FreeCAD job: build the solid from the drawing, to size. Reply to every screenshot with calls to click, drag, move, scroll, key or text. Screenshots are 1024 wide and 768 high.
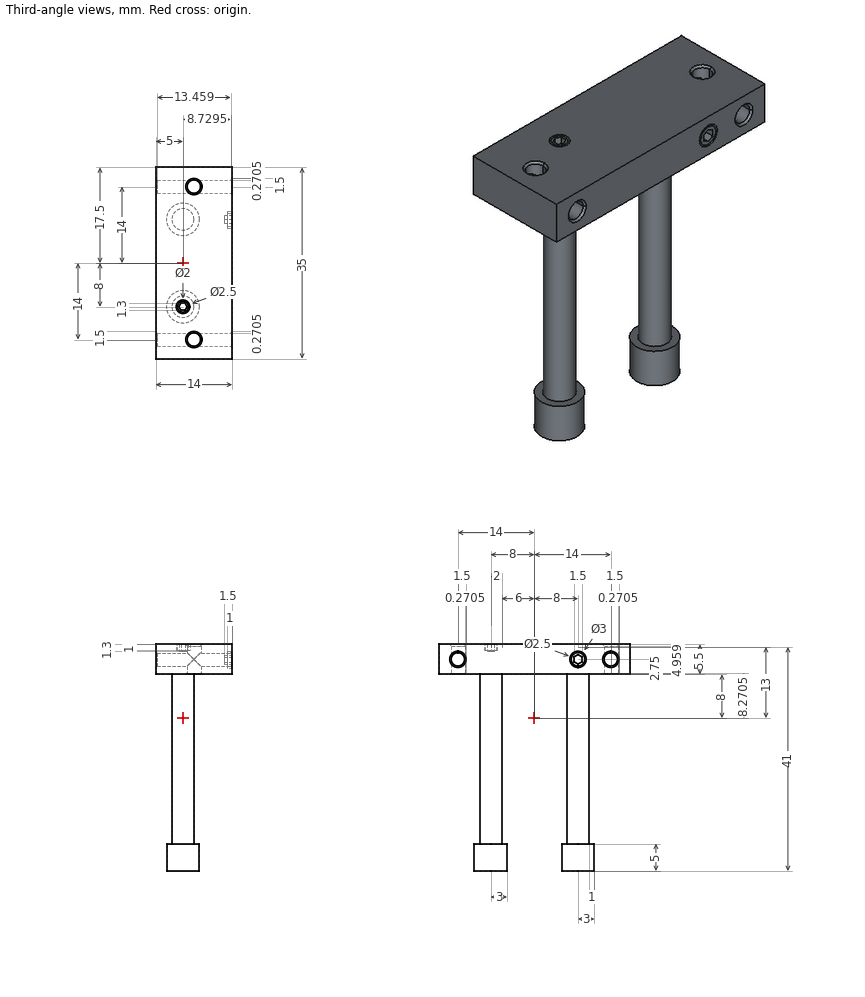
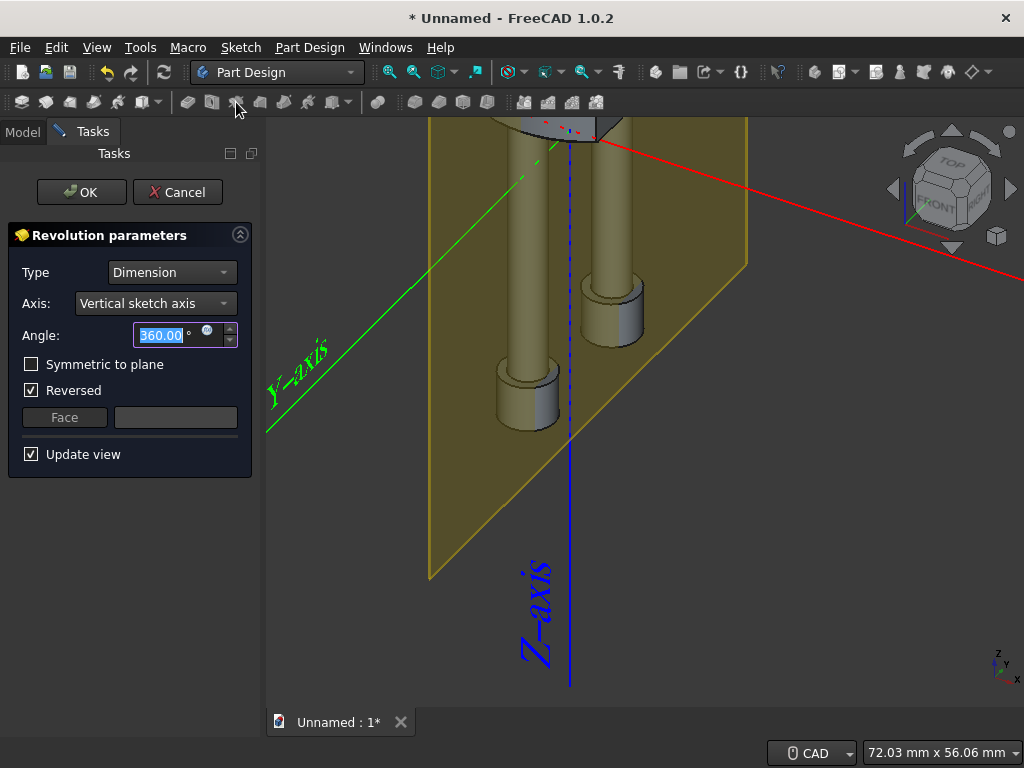
click(156, 304)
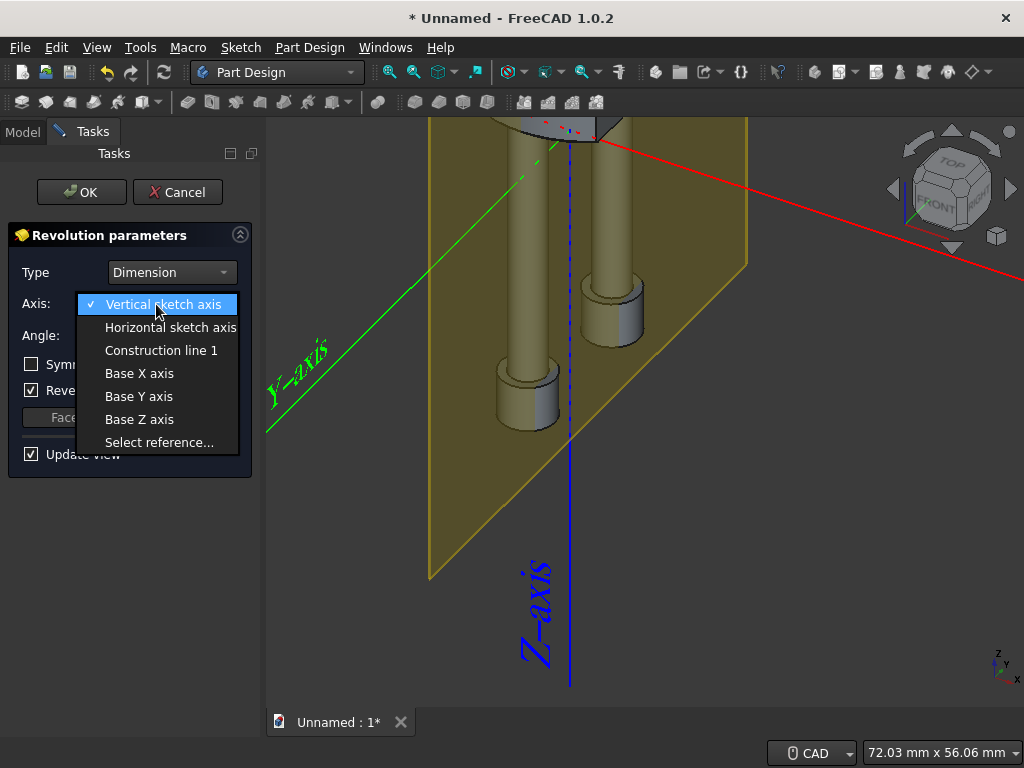
click(156, 350)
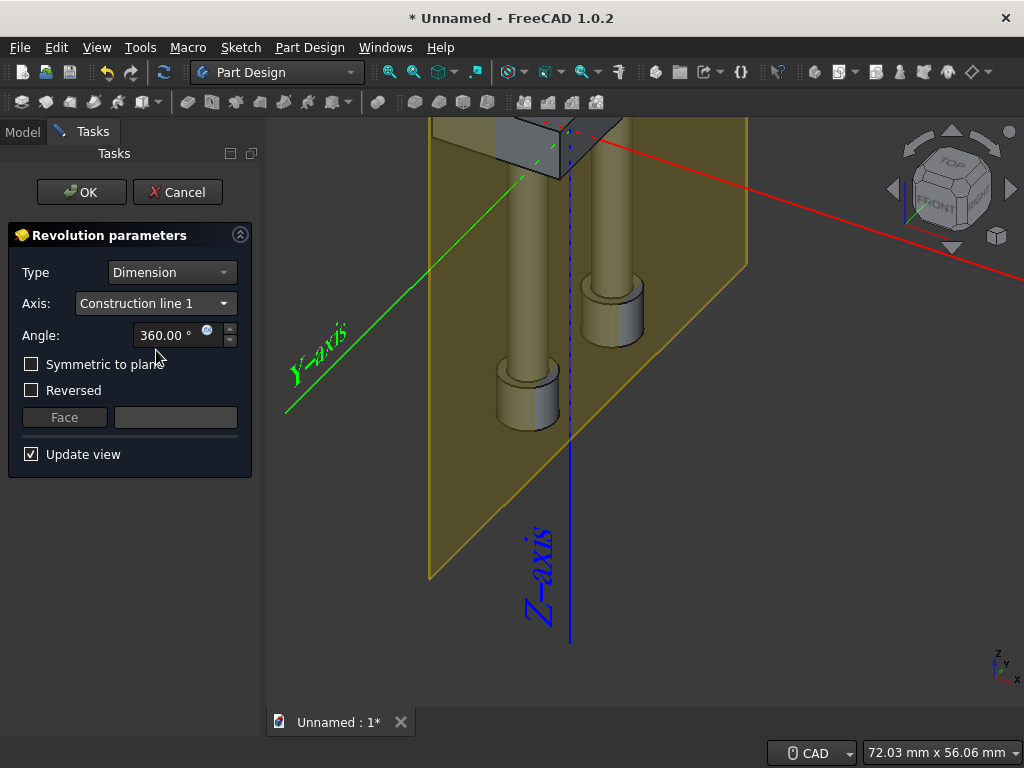
click(82, 192)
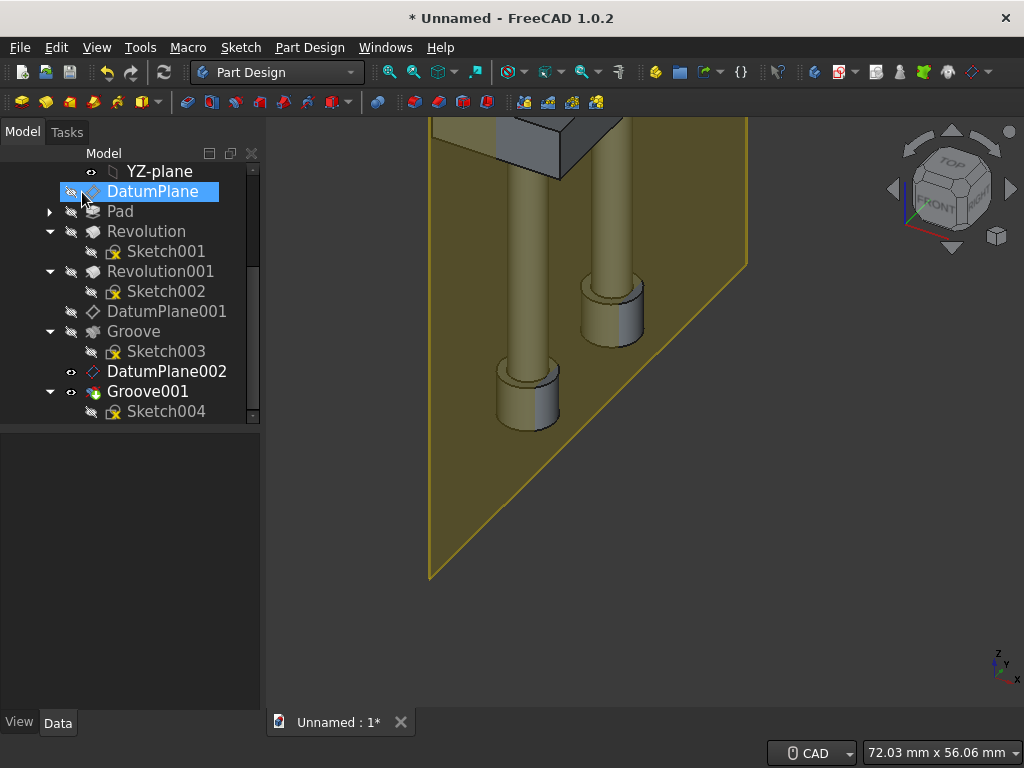
click(116, 372)
key(space)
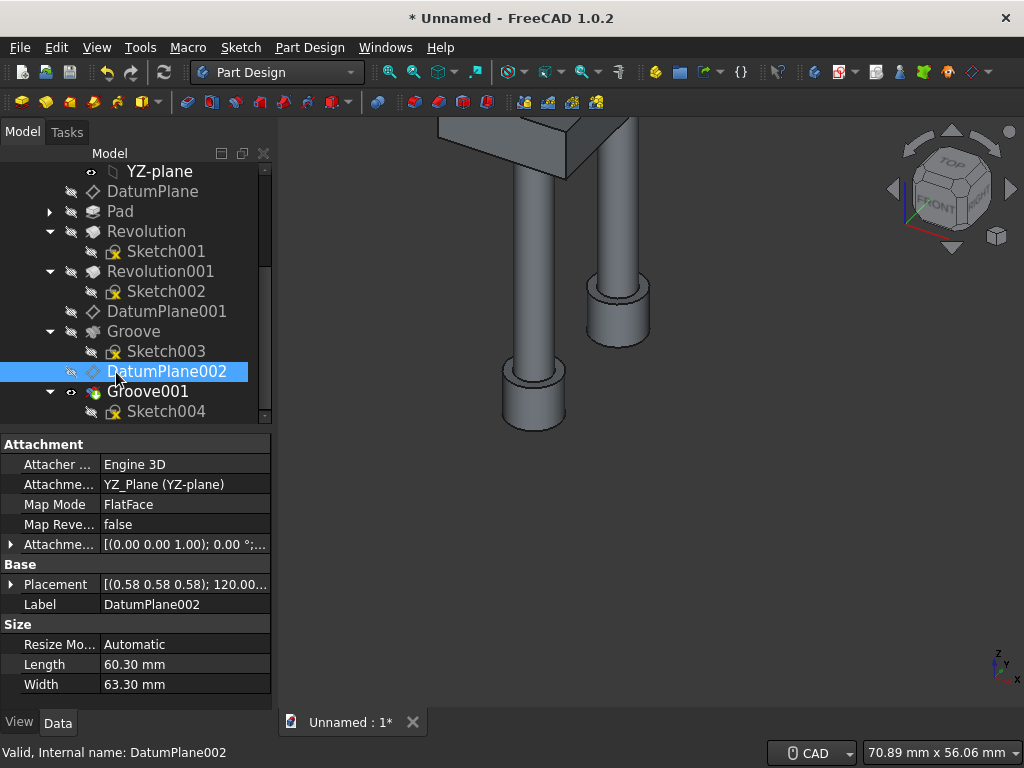
click(390, 72)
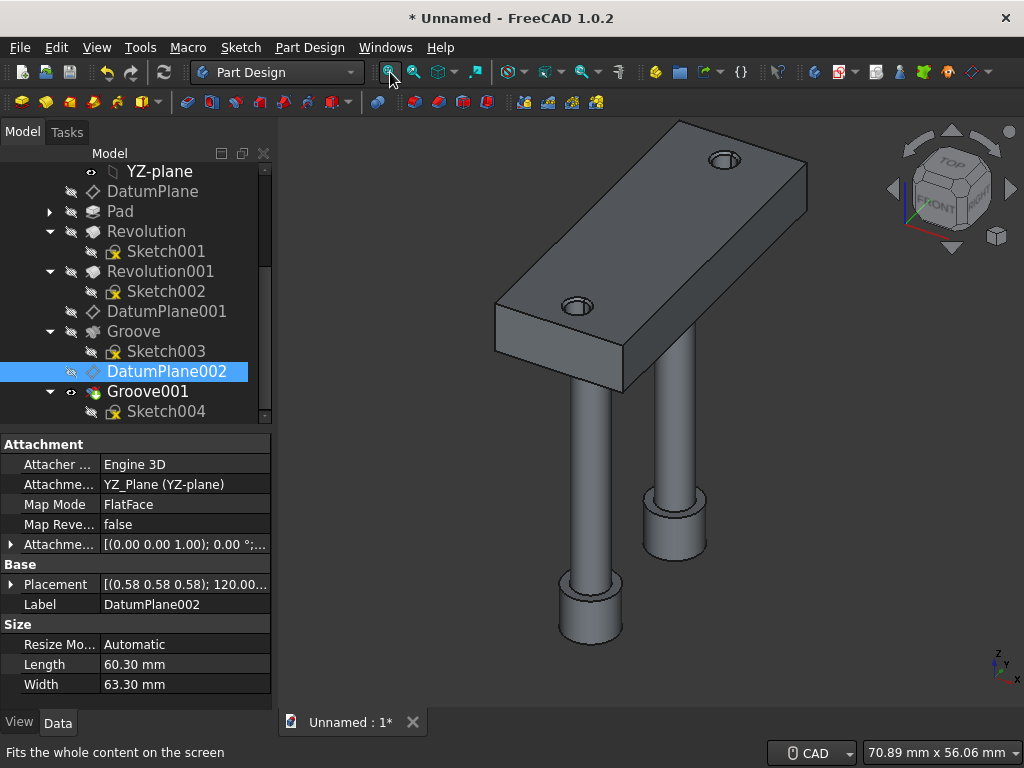
scroll(160, 287, down, 3)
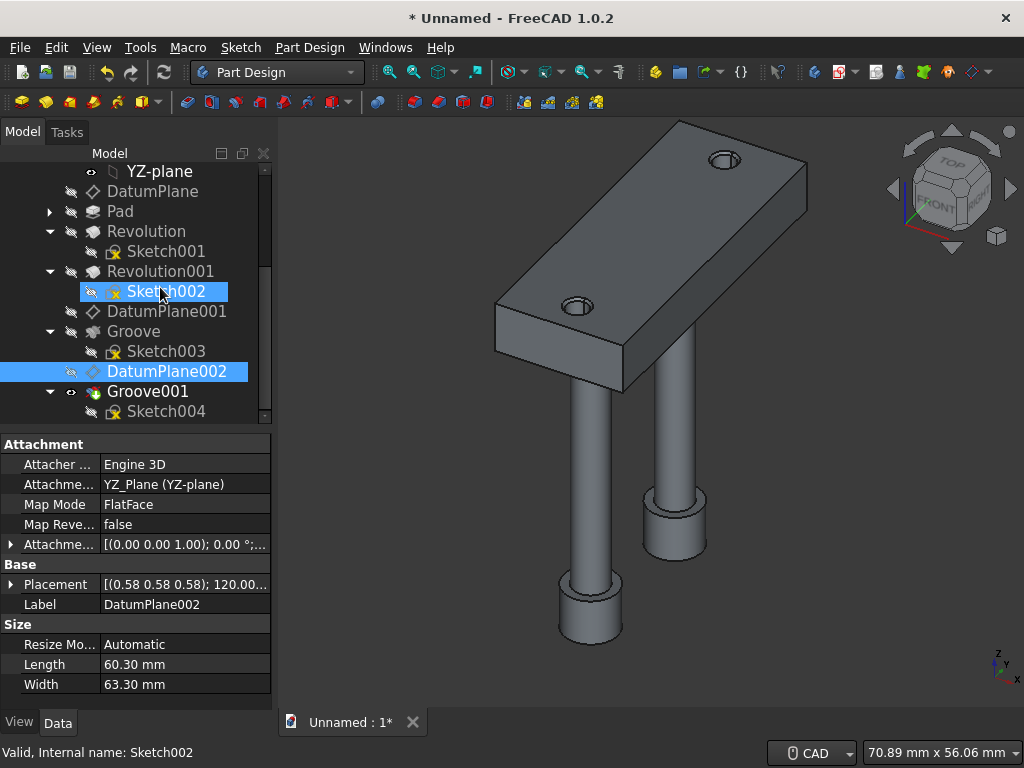
scroll(160, 287, up, 15)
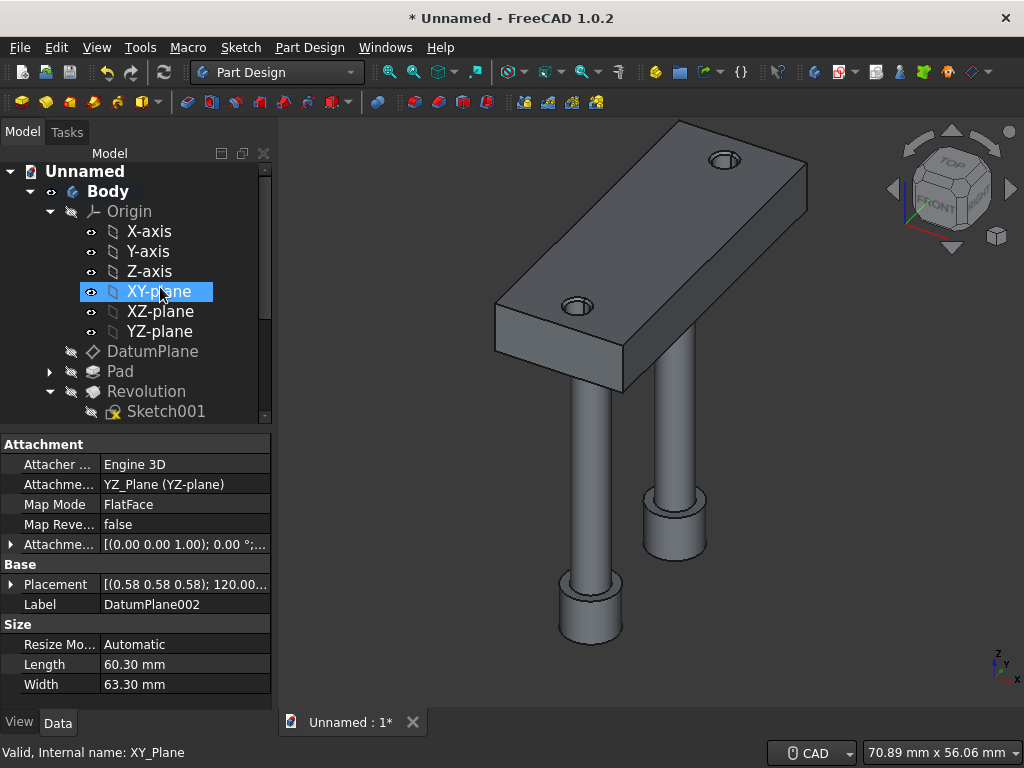
click(136, 292)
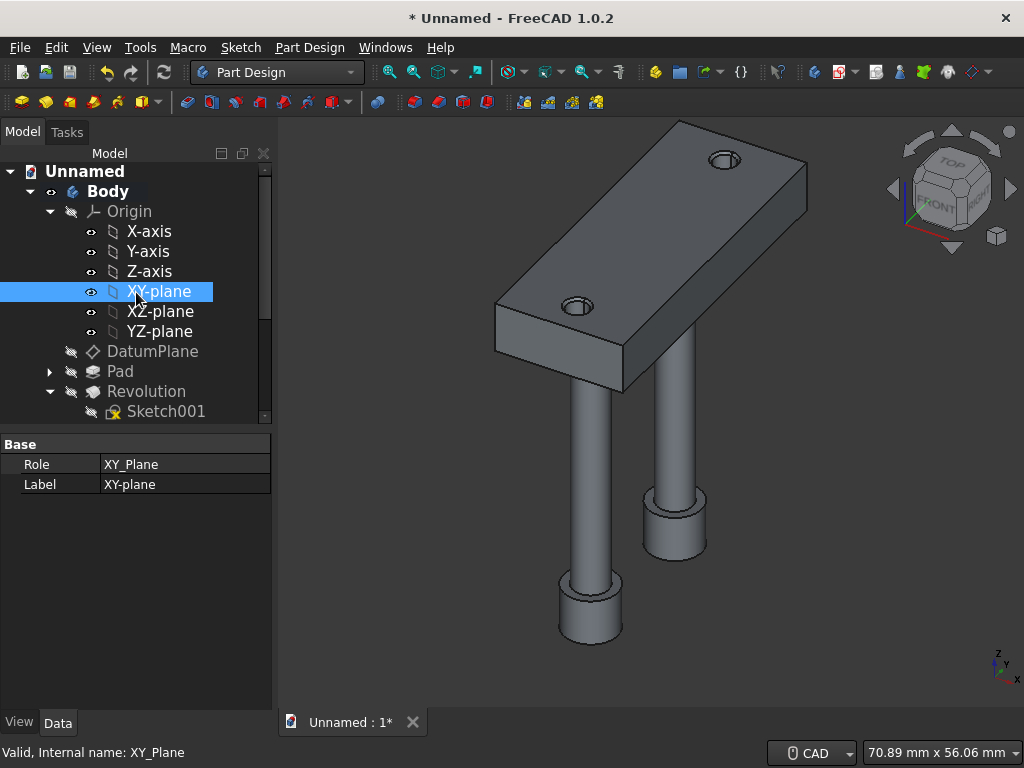
click(972, 72)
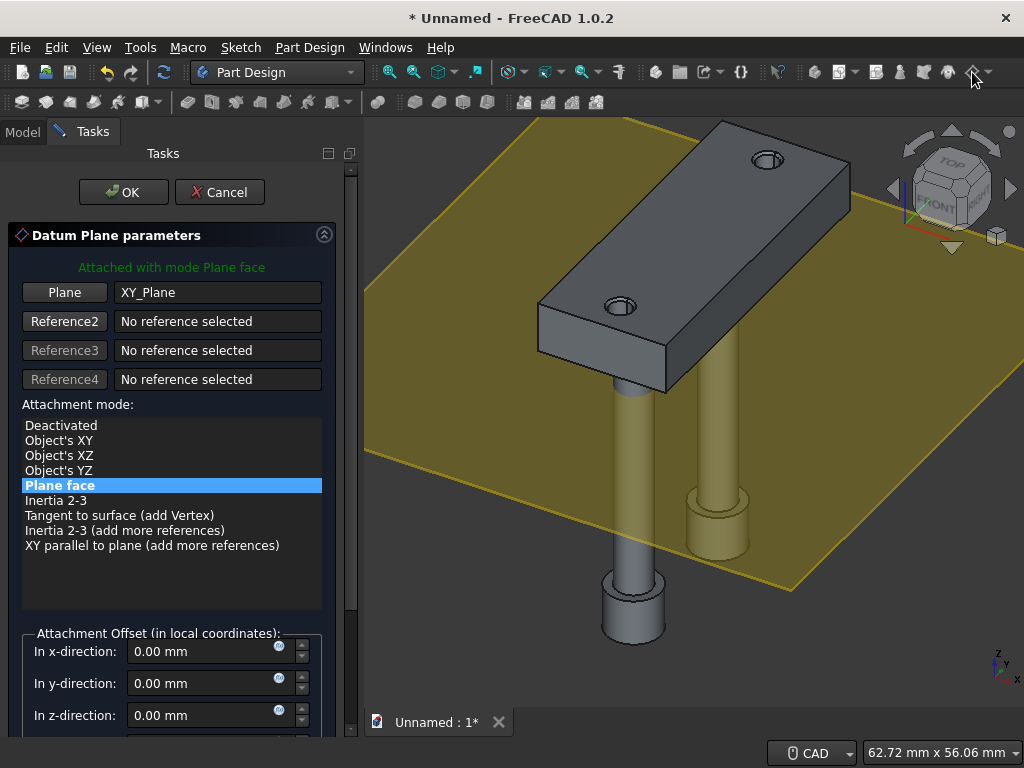
triple_click(210, 715)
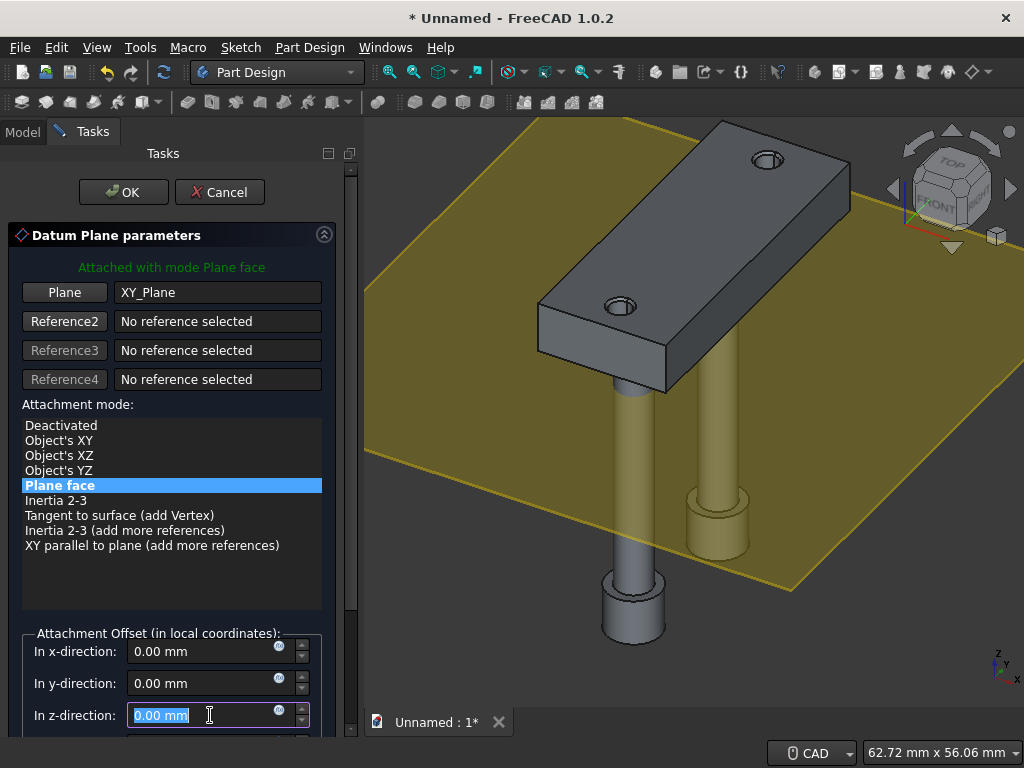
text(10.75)
key(Tab)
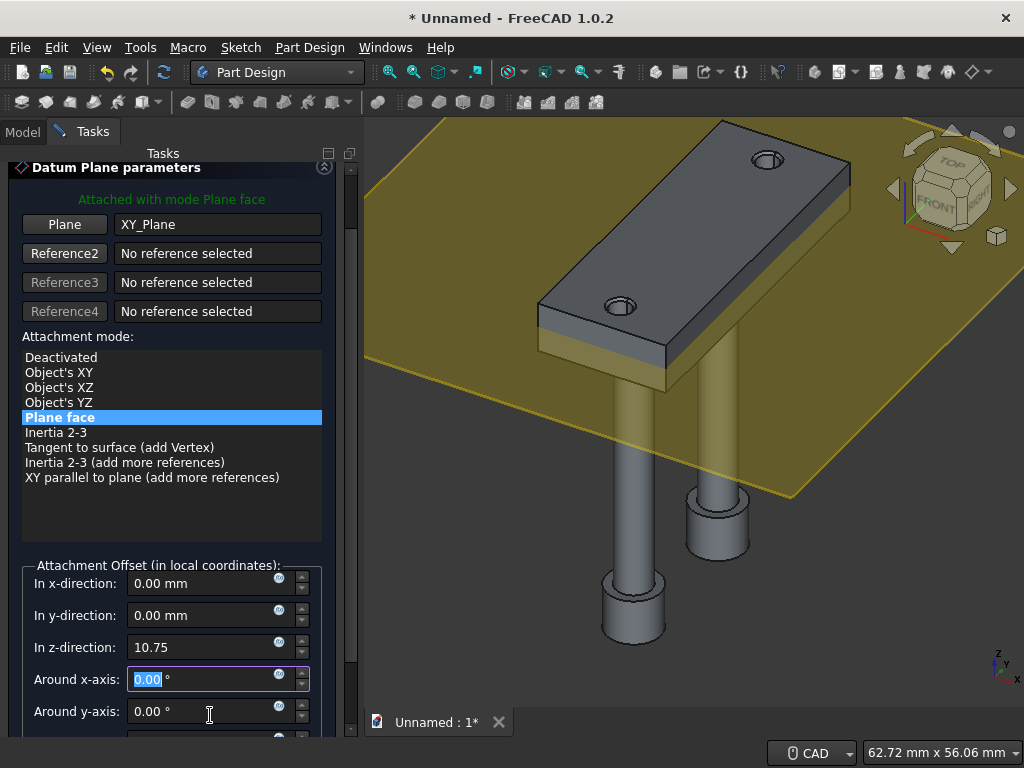
scroll(351, 450, up, 2)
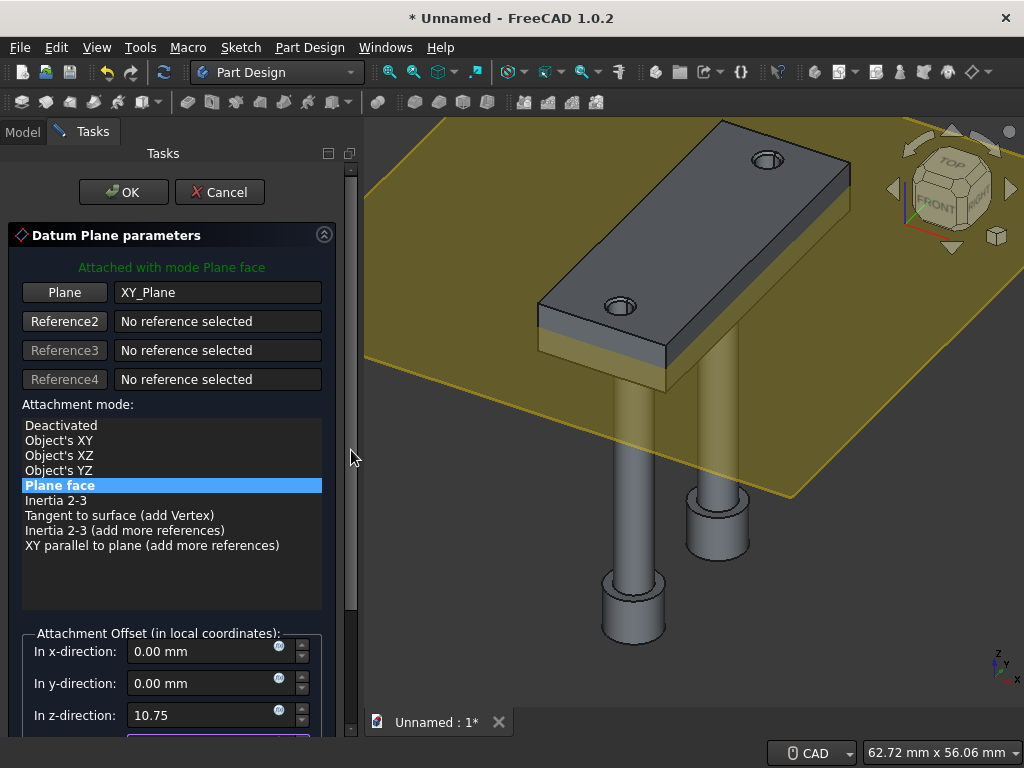
click(124, 192)